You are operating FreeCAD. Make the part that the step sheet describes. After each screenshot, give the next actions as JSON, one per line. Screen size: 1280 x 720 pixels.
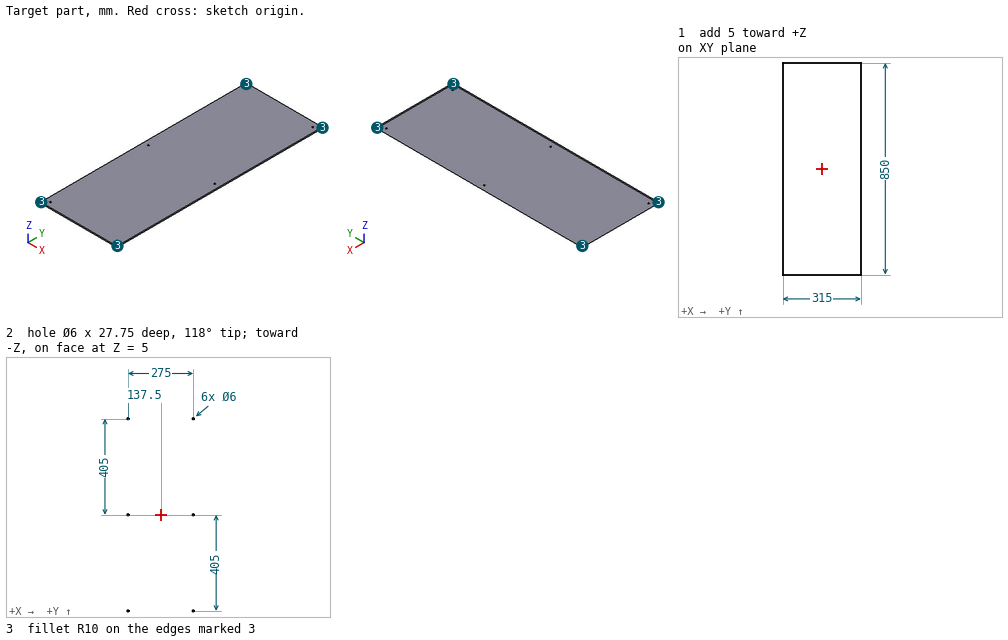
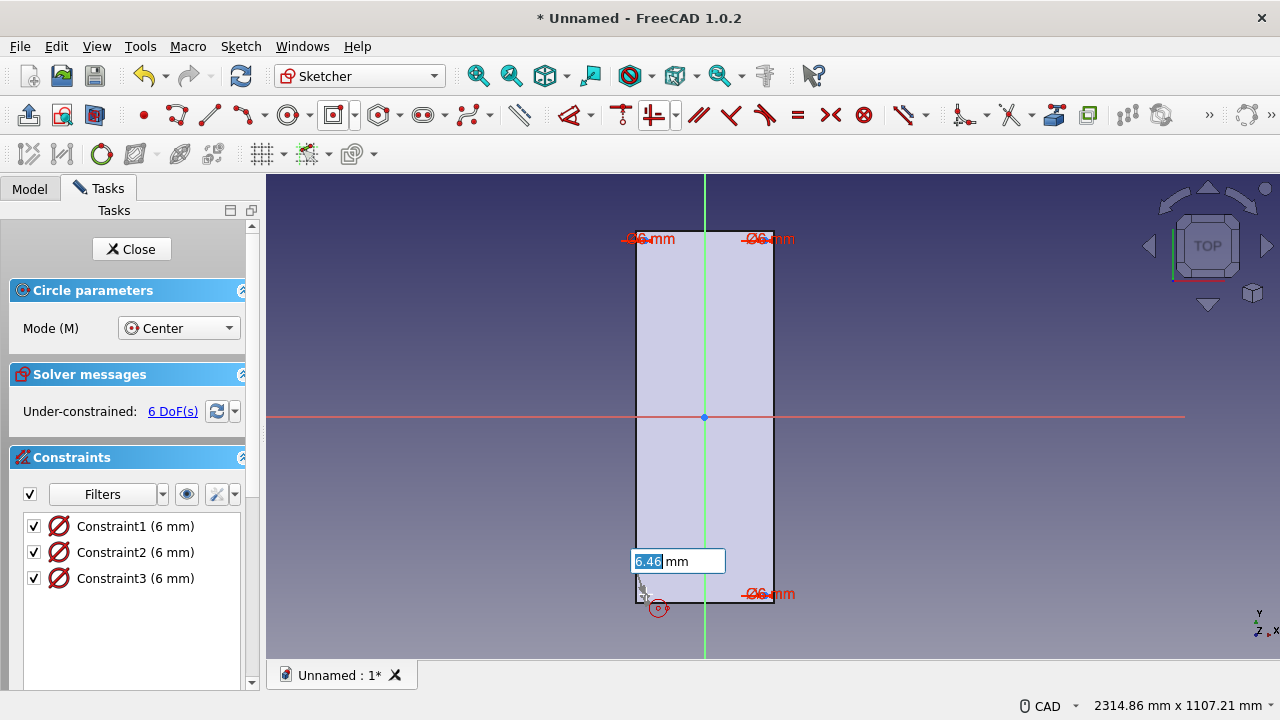
{"action": "type", "text": "6"}
{"action": "key", "text": "Return"}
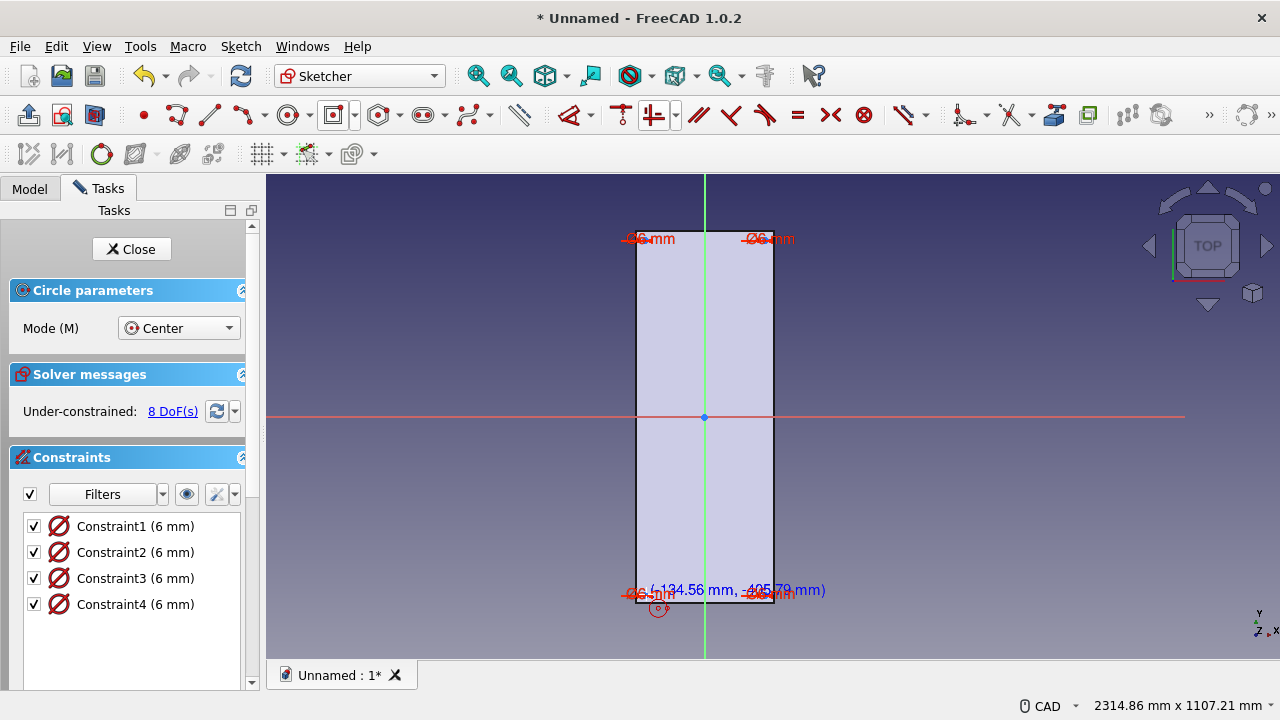
{"action": "scroll", "coordinate": [645, 417], "scroll_direction": "up", "scroll_amount": 15}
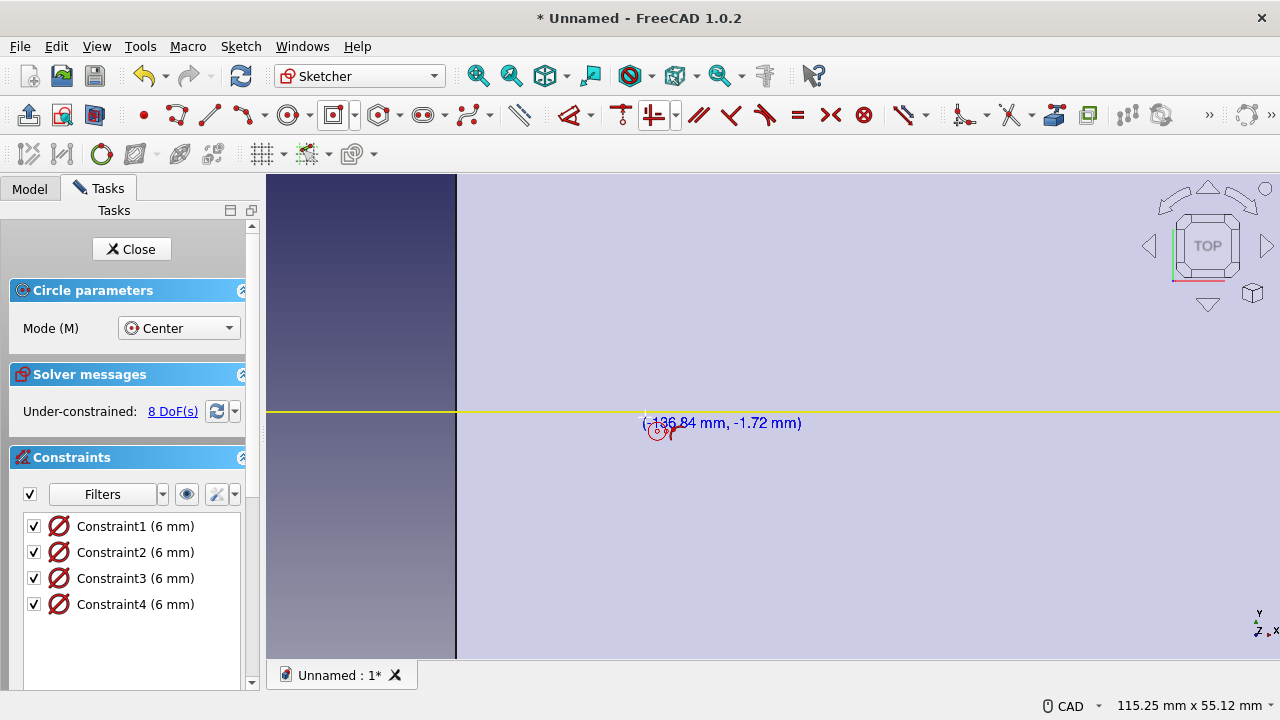
{"action": "scroll", "coordinate": [645, 417], "scroll_direction": "down", "scroll_amount": 15}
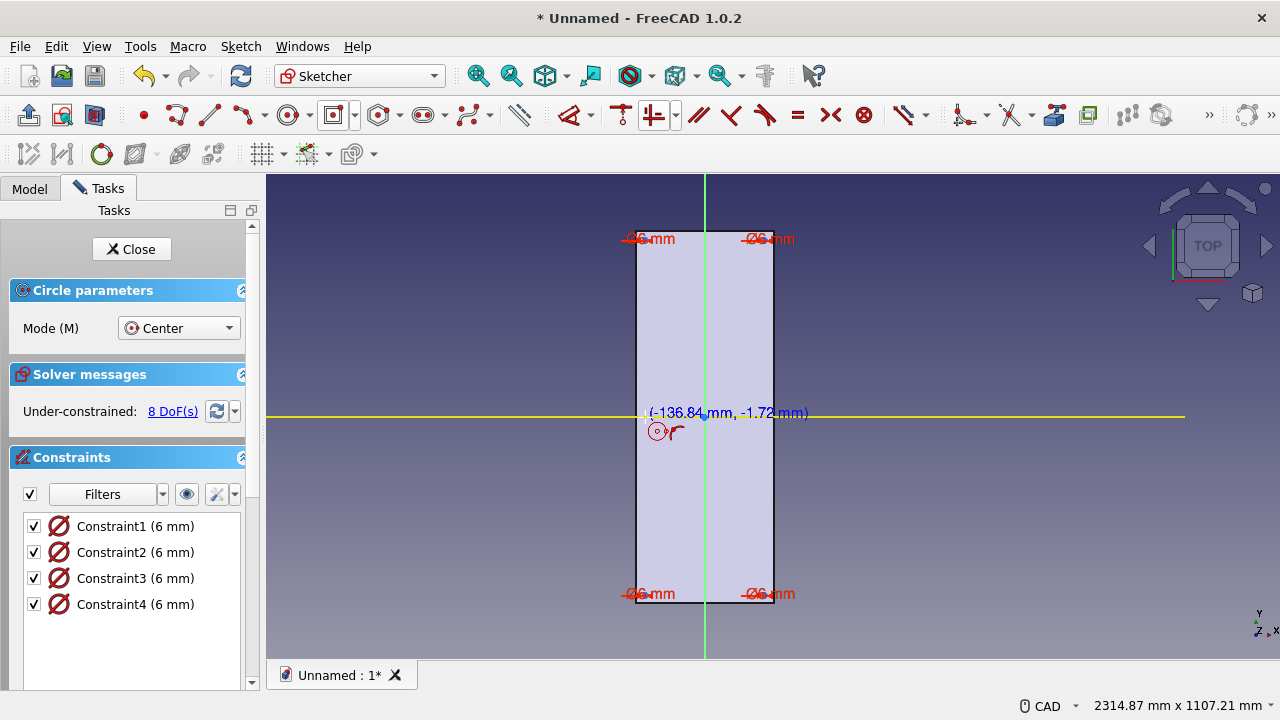
{"action": "left_click", "coordinate": [645, 417]}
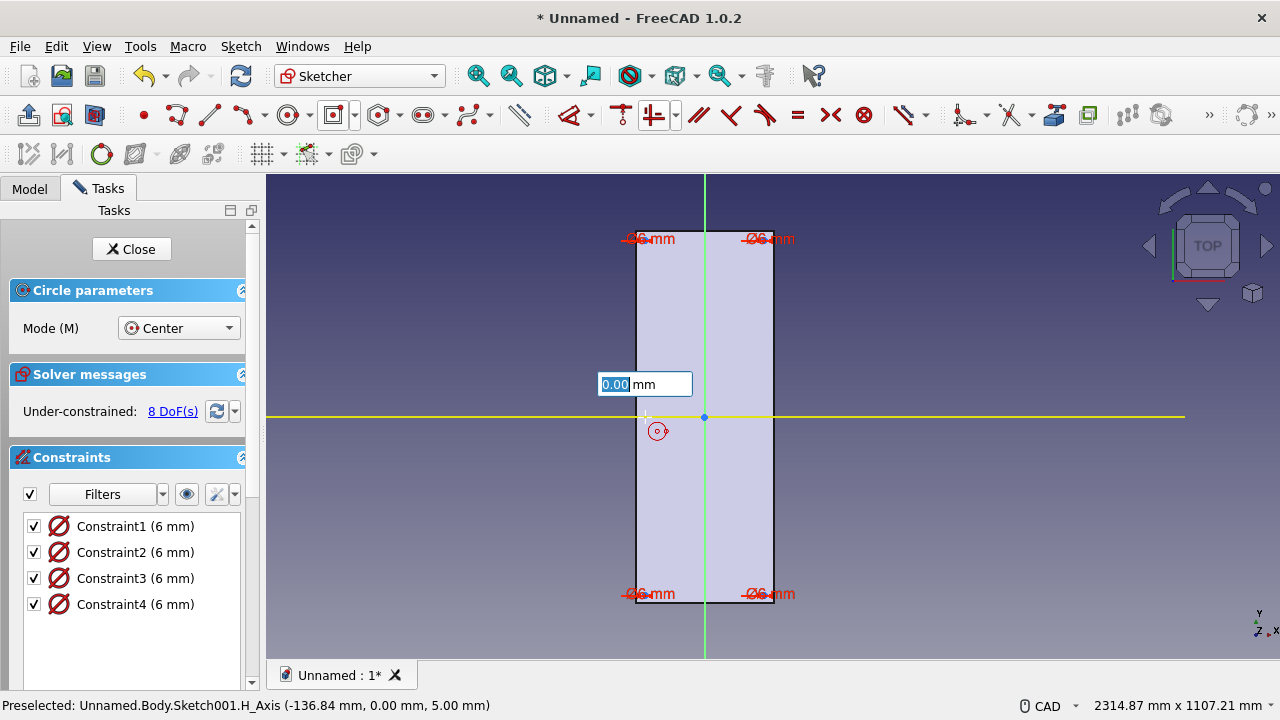
{"action": "scroll", "coordinate": [644, 418], "scroll_direction": "up", "scroll_amount": 13}
{"action": "mouse_move", "coordinate": [643, 418]}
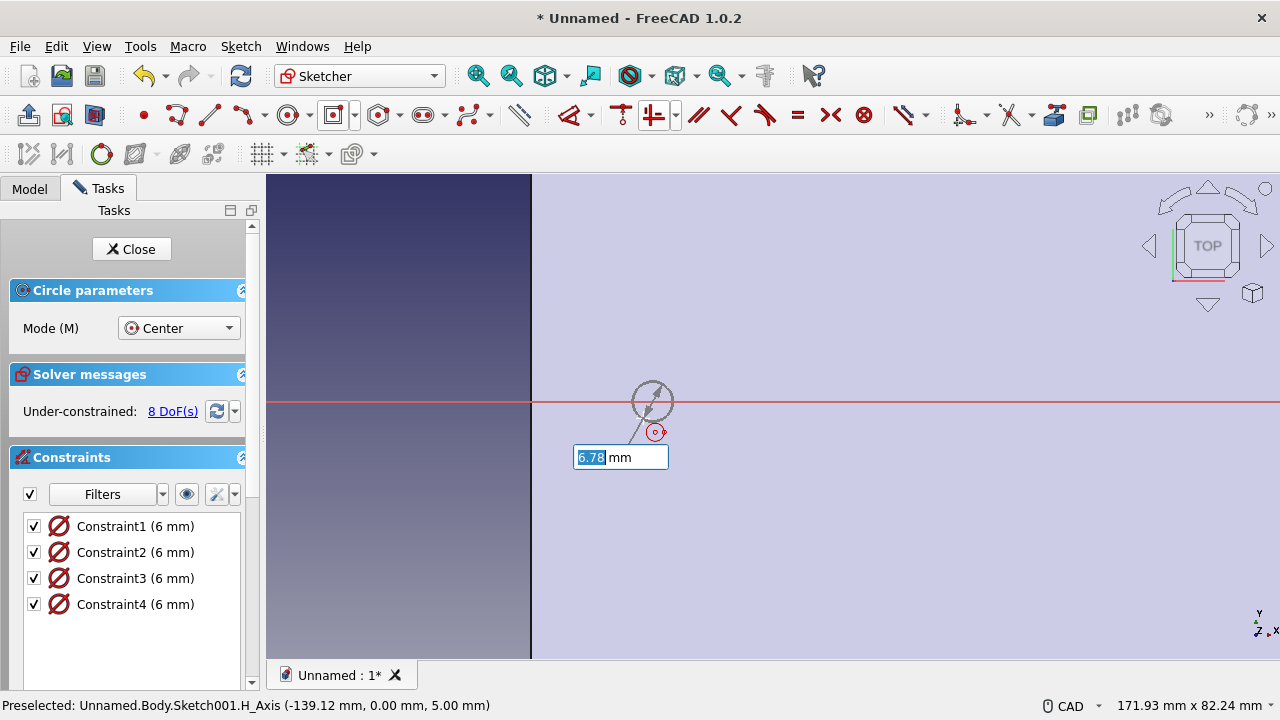
{"action": "type", "text": "6"}
{"action": "key", "text": "Return"}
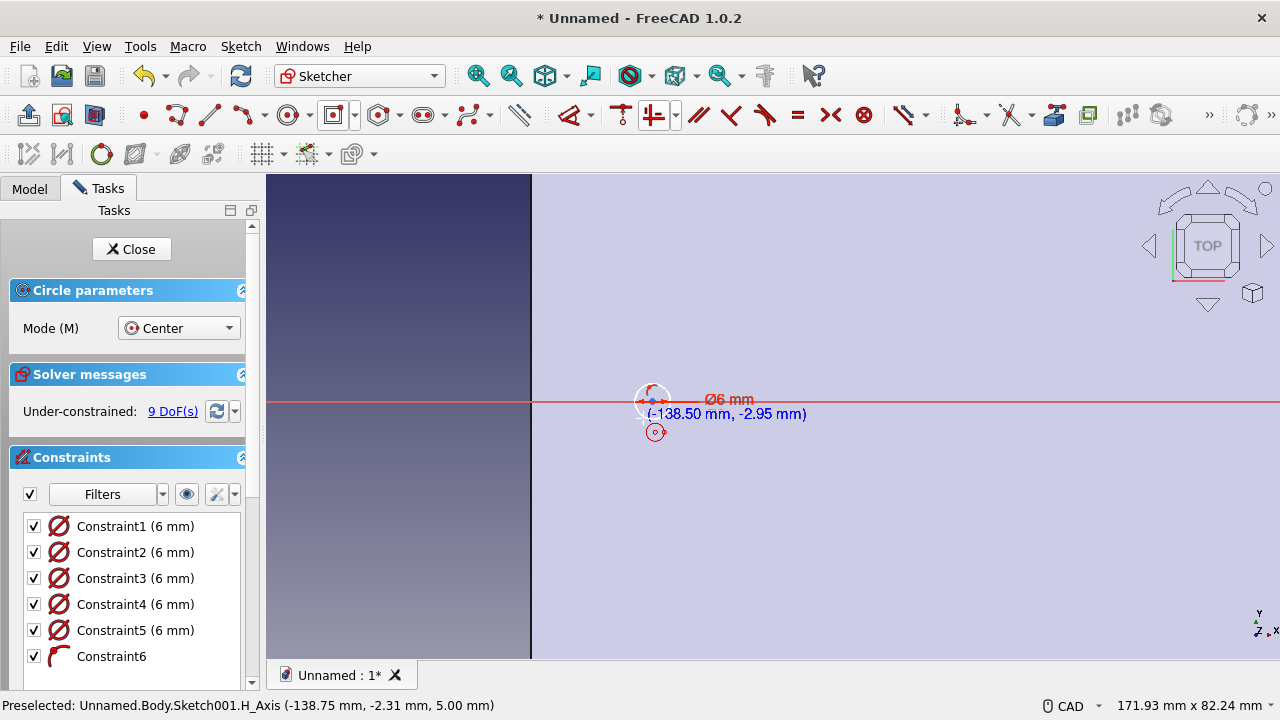
{"action": "scroll", "coordinate": [656, 417], "scroll_direction": "down", "scroll_amount": 14}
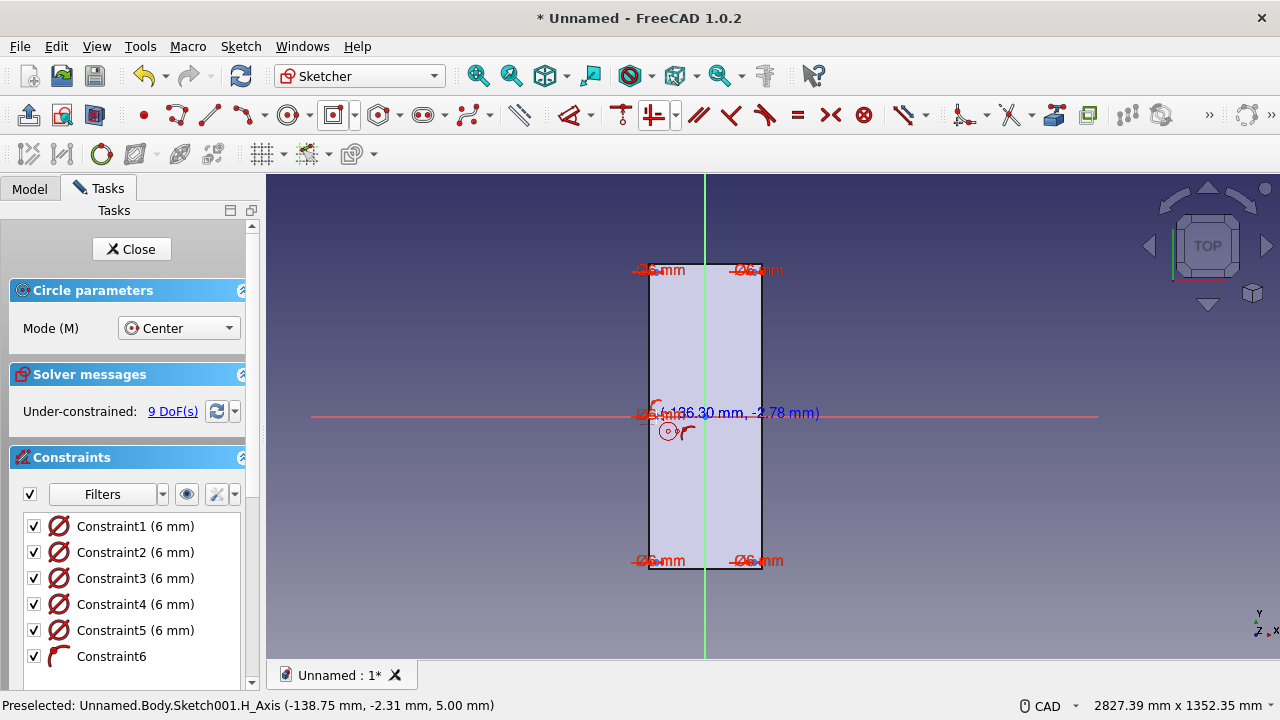
{"action": "scroll", "coordinate": [755, 417], "scroll_direction": "up", "scroll_amount": 16}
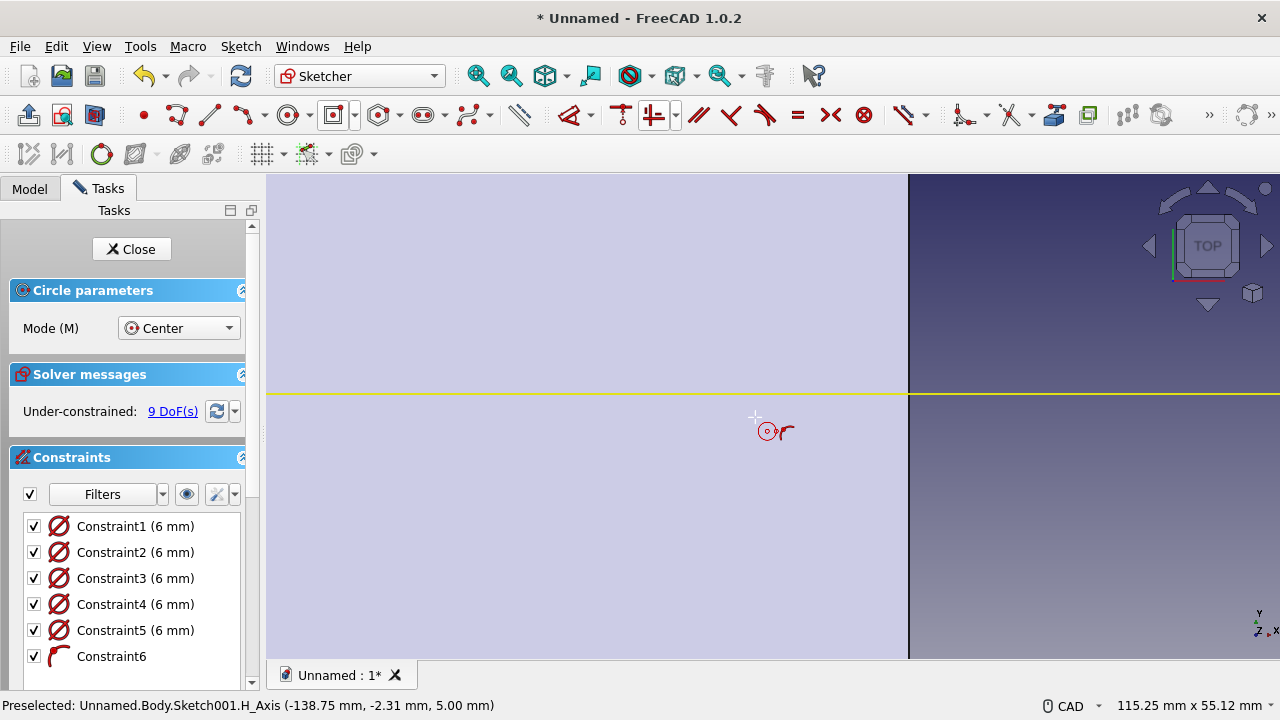
{"action": "scroll", "coordinate": [766, 418], "scroll_direction": "down", "scroll_amount": 15}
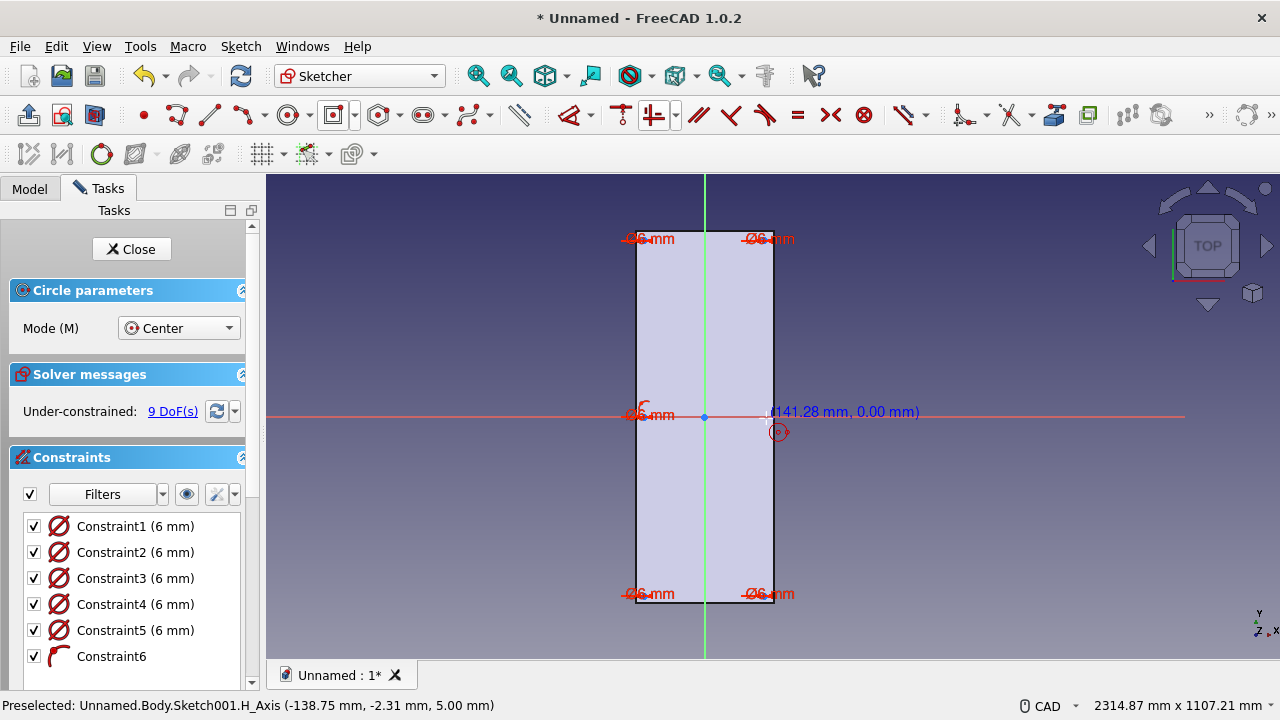
{"action": "left_click", "coordinate": [765, 417]}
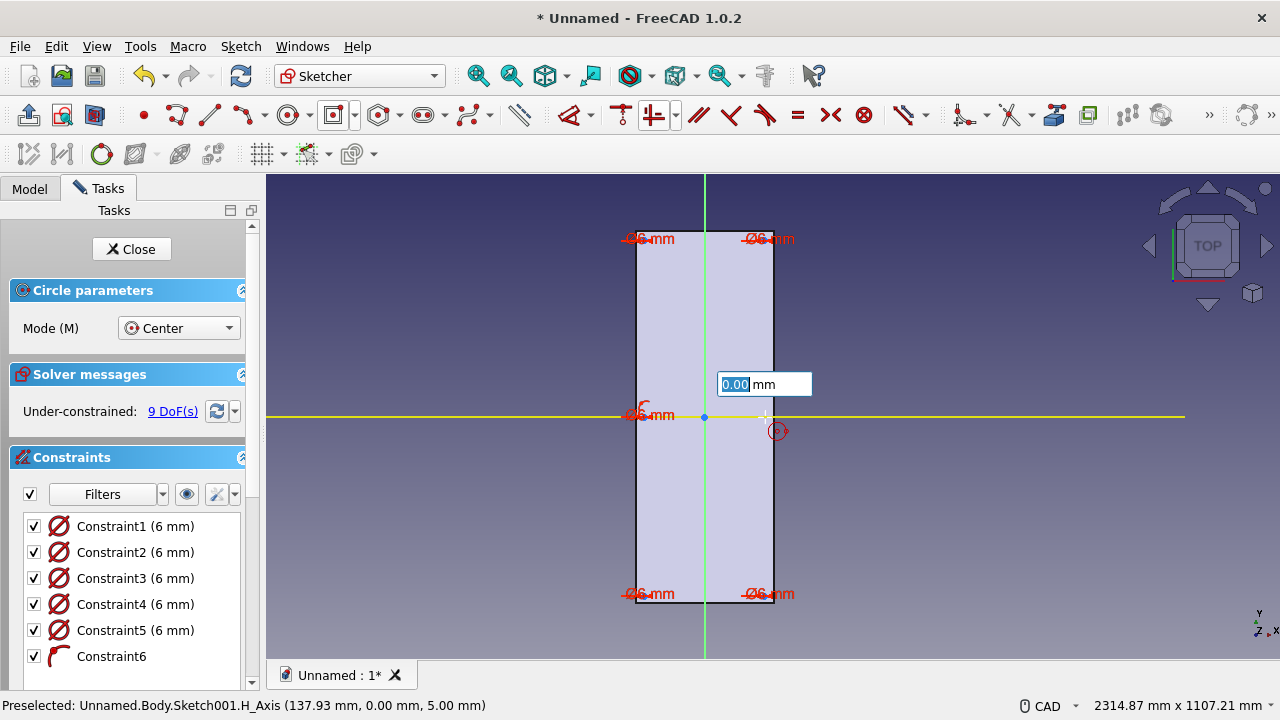
{"action": "scroll", "coordinate": [764, 419], "scroll_direction": "up", "scroll_amount": 13}
{"action": "mouse_move", "coordinate": [763, 406]}